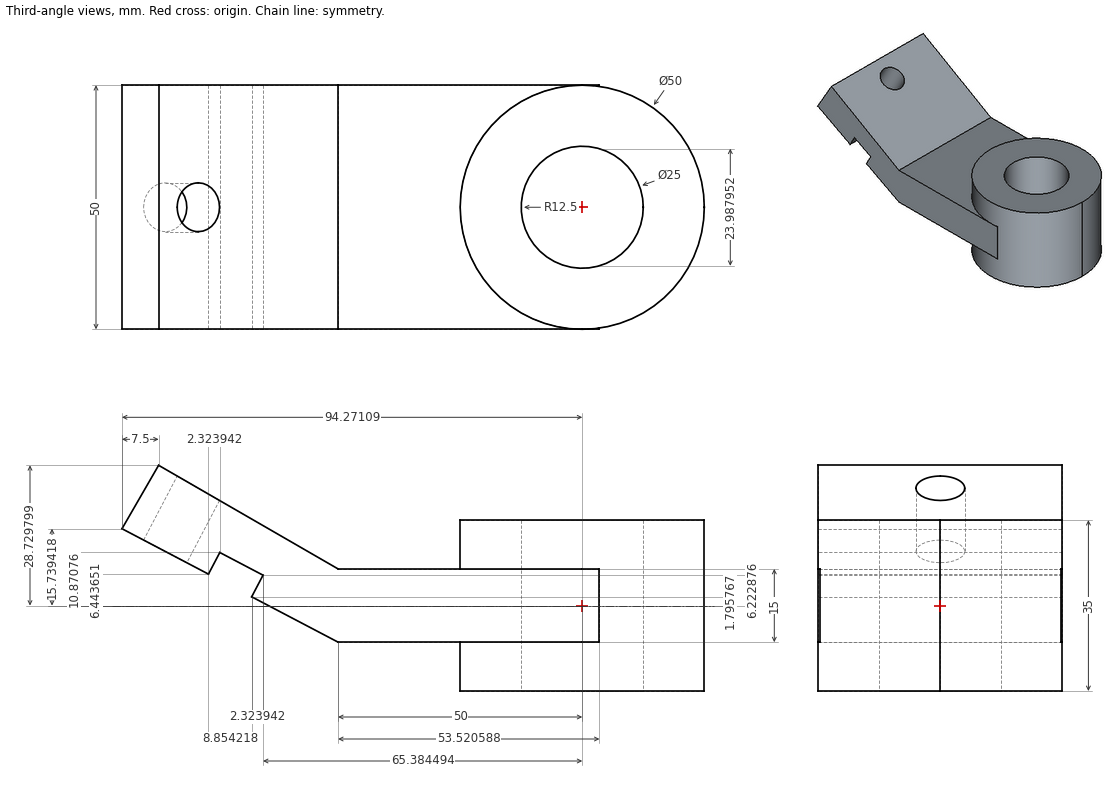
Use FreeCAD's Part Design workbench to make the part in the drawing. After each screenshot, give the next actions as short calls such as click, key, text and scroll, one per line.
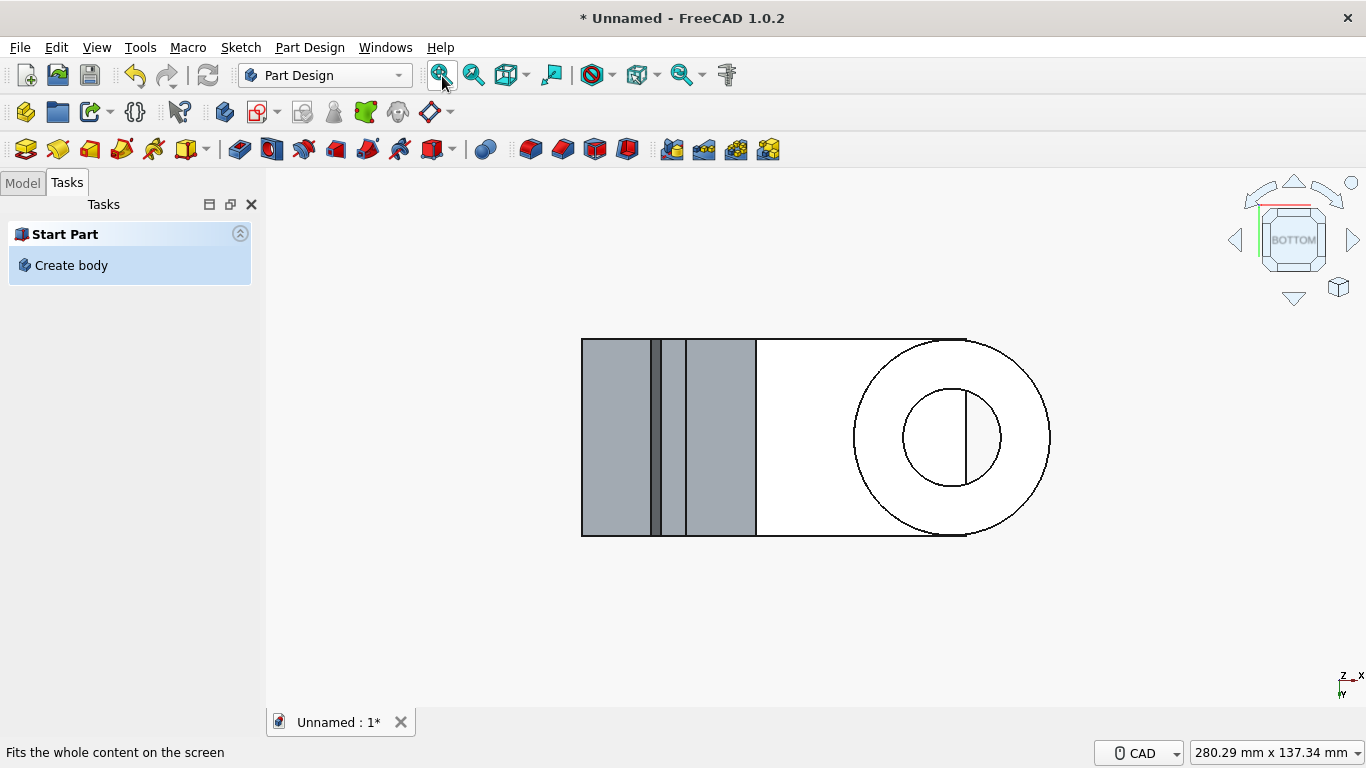
click(721, 493)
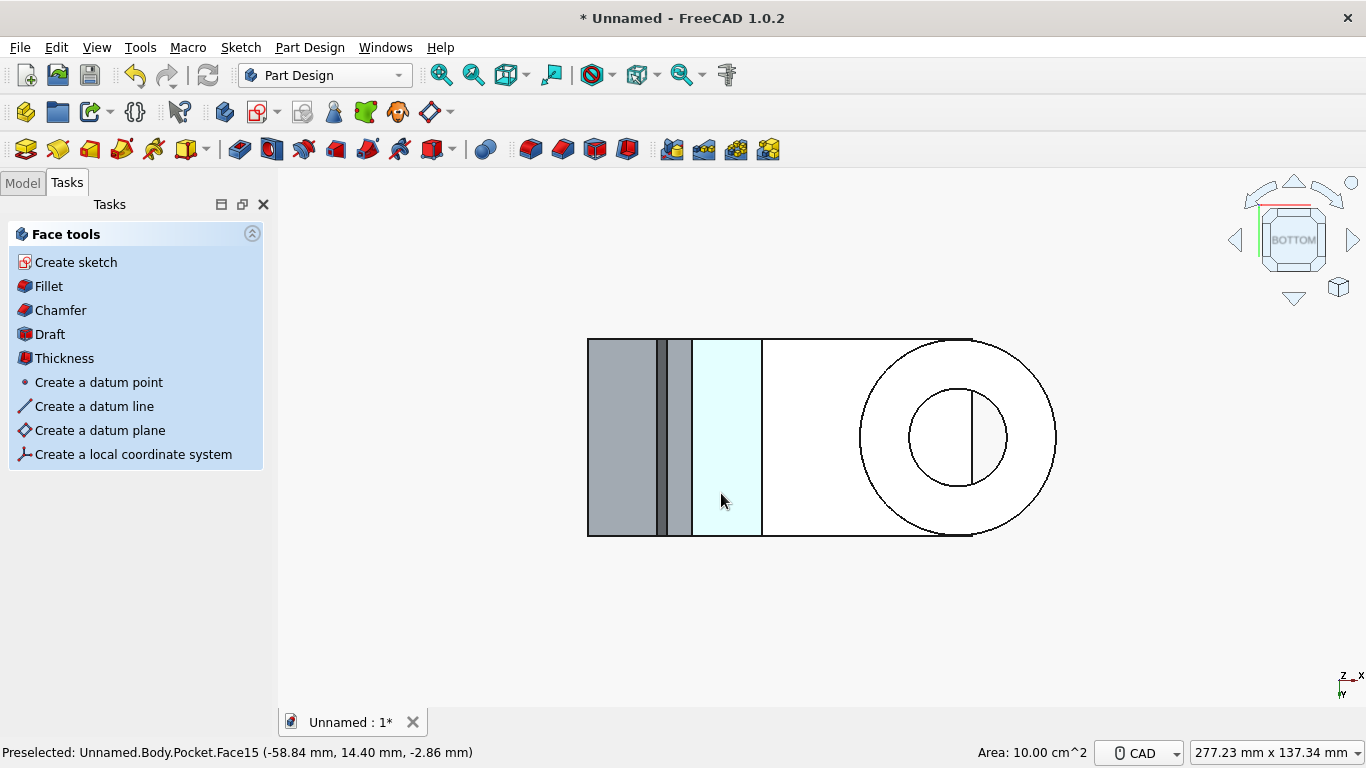
click(258, 112)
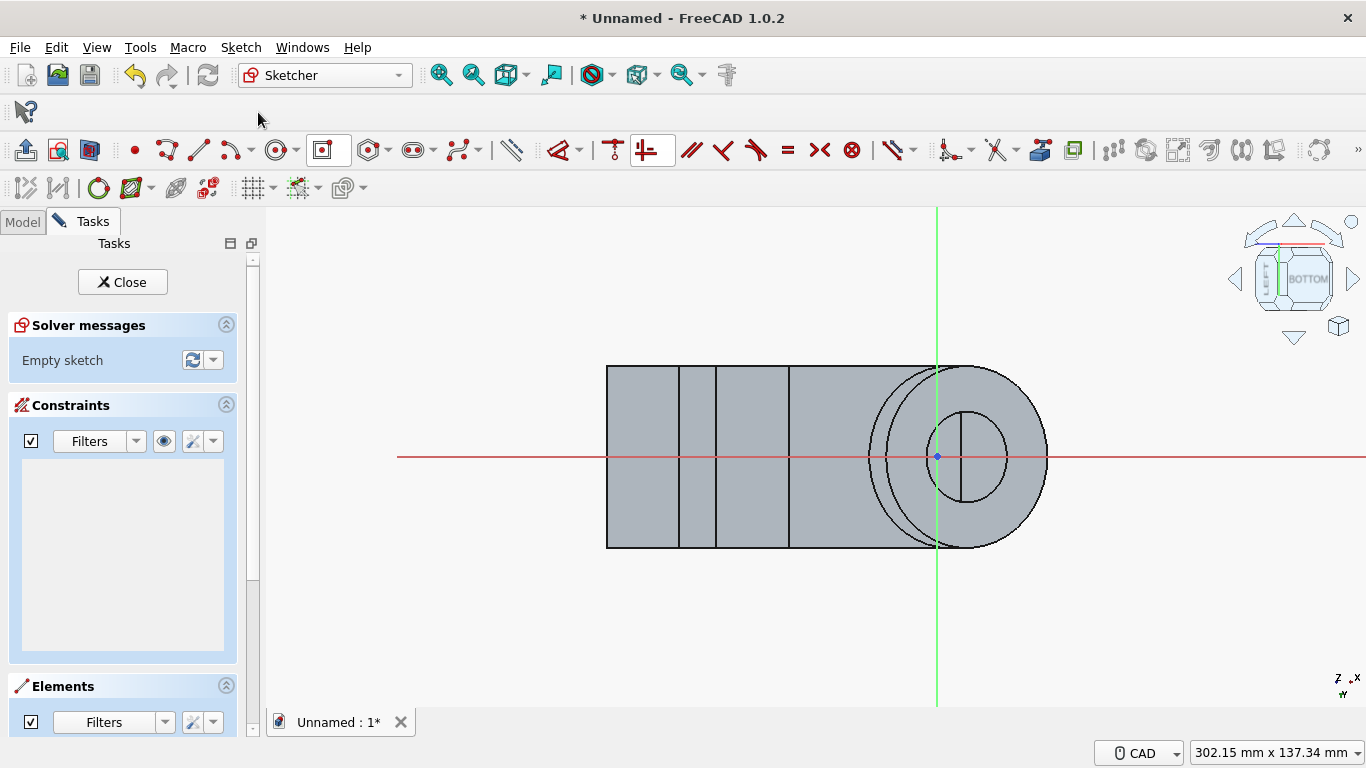
scroll(630, 457, up, 11)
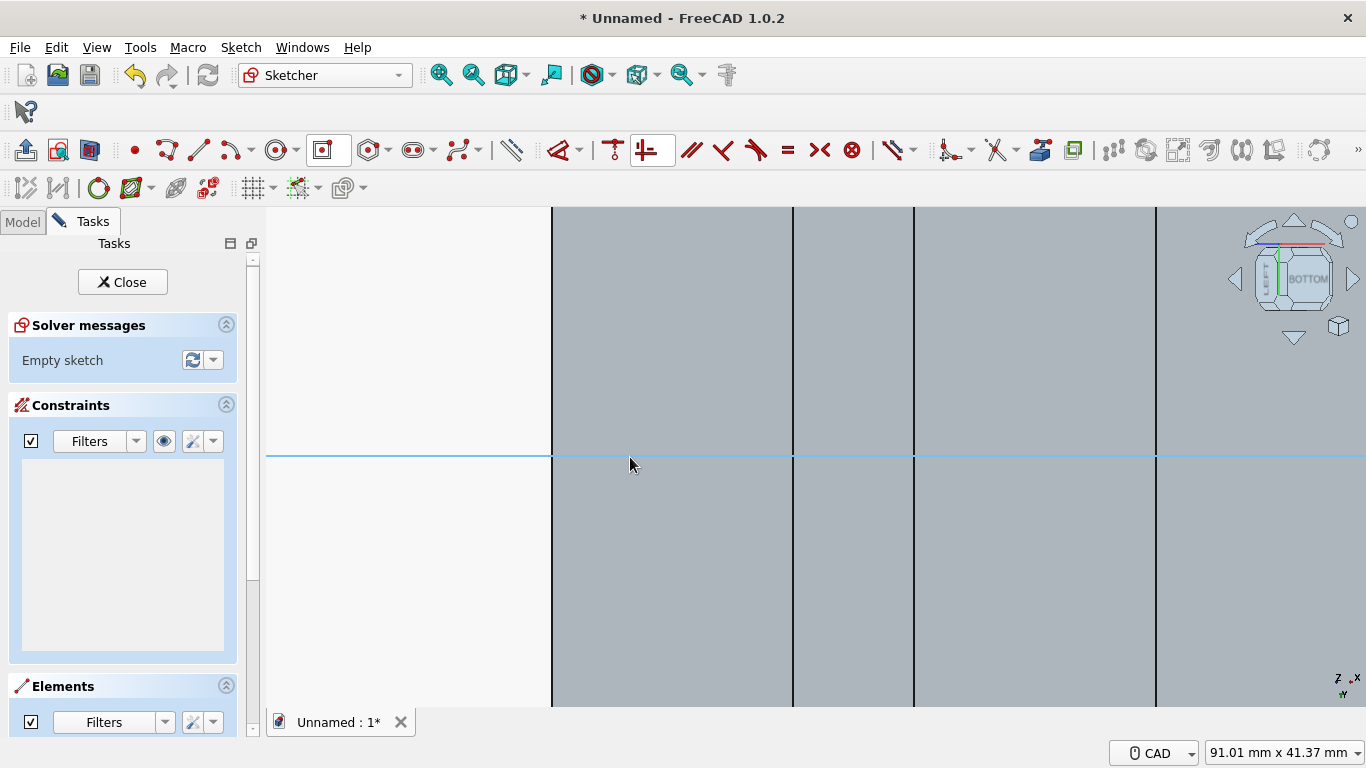
click(276, 150)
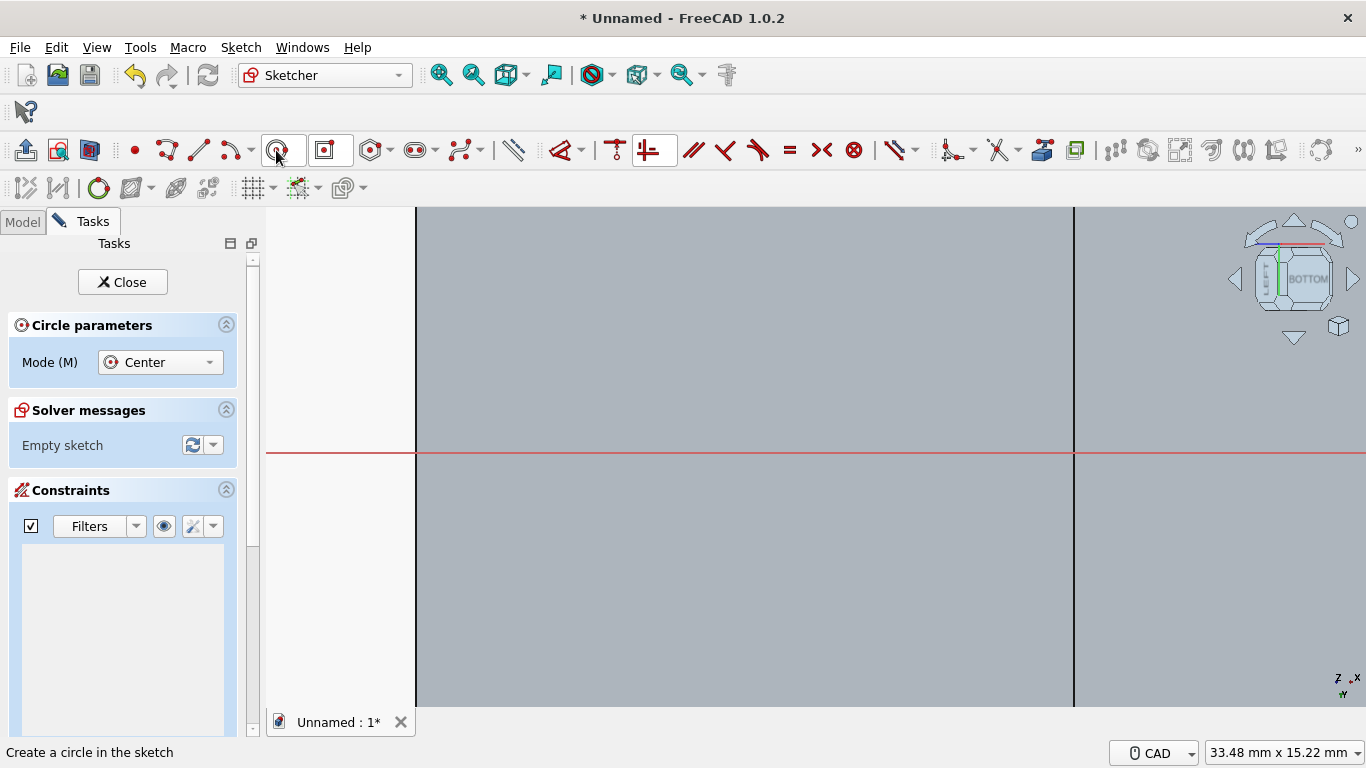
click(745, 453)
click(861, 337)
key(Escape)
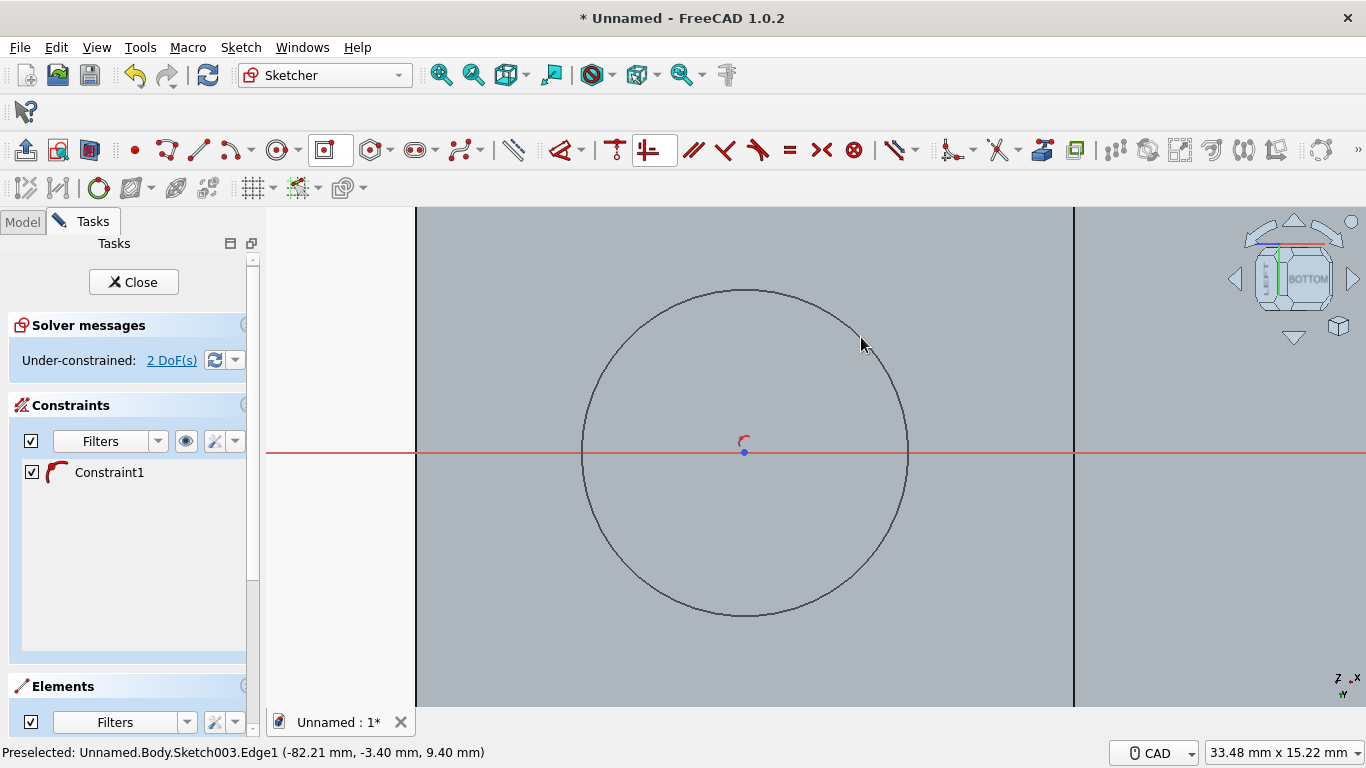
click(560, 150)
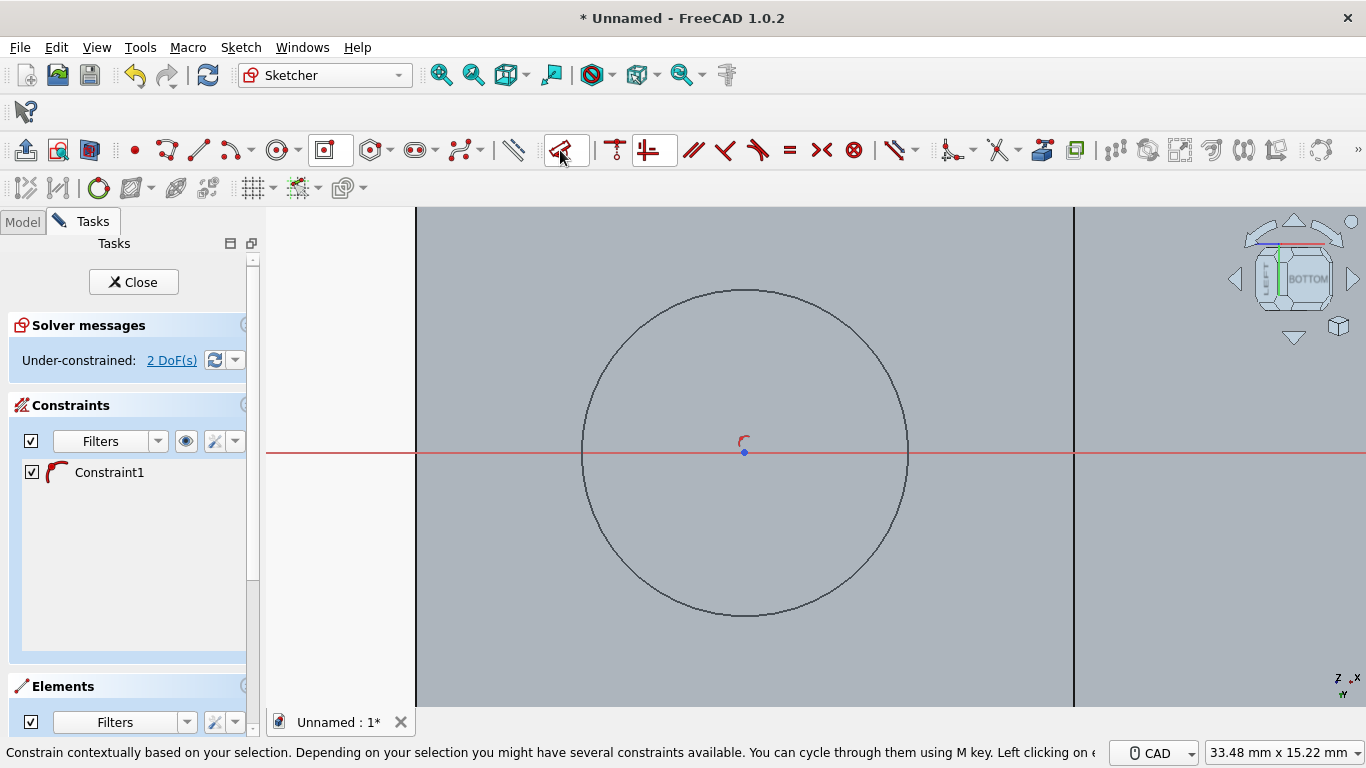
click(860, 337)
click(883, 314)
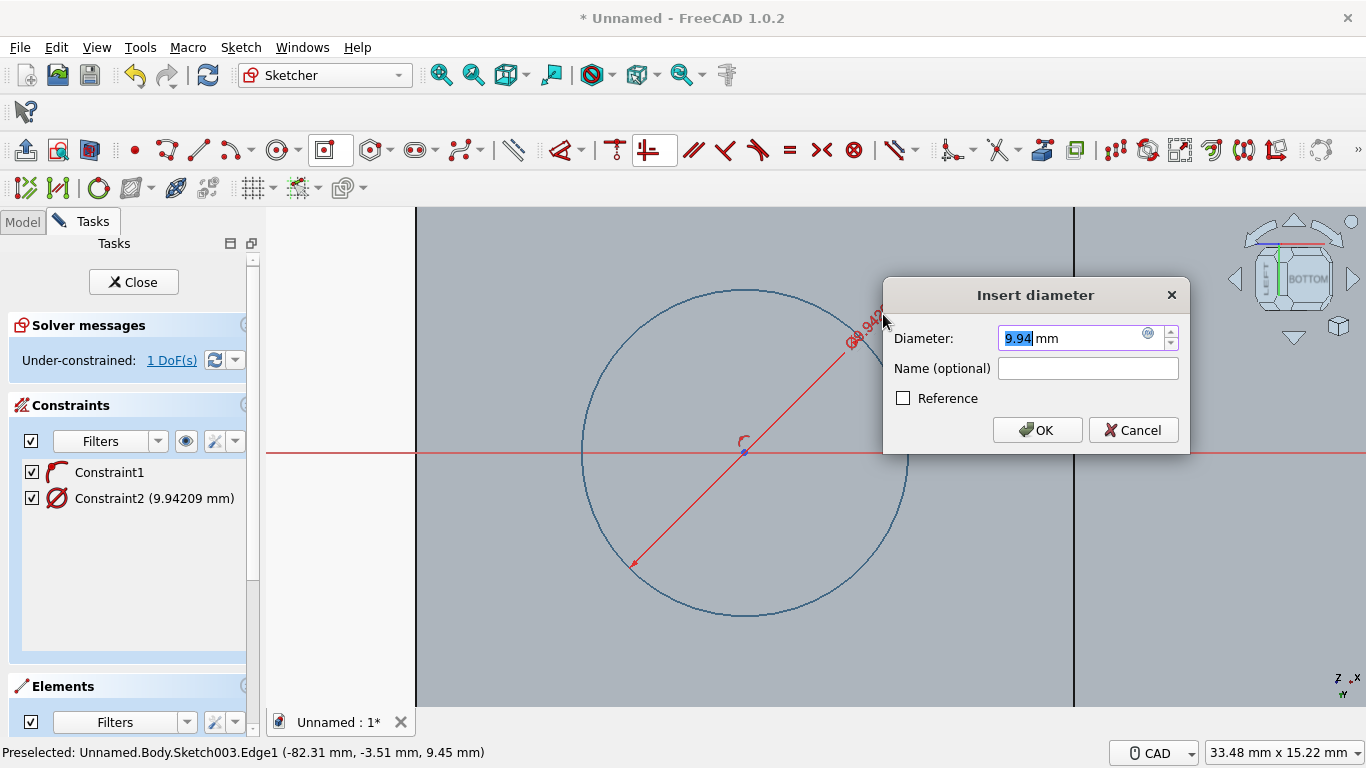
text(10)
key(Return)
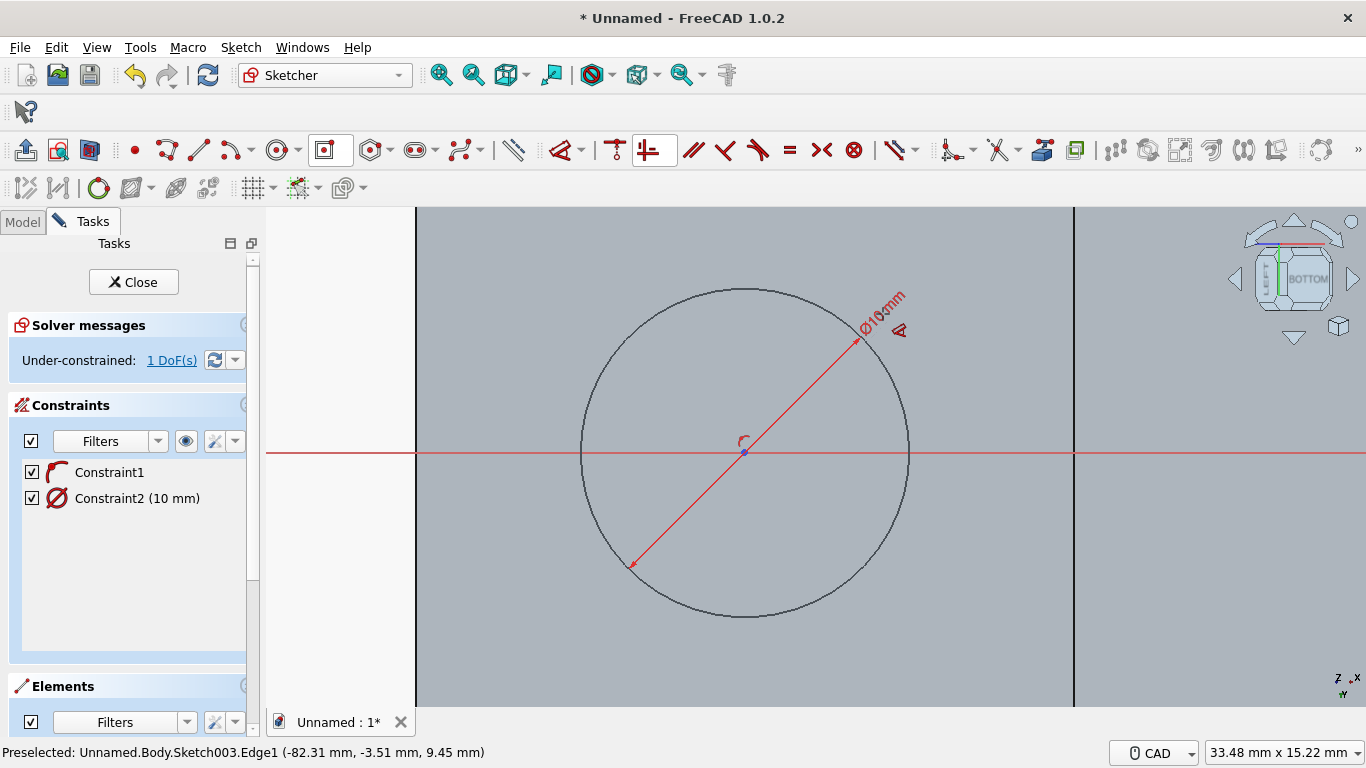
click(745, 453)
click(973, 487)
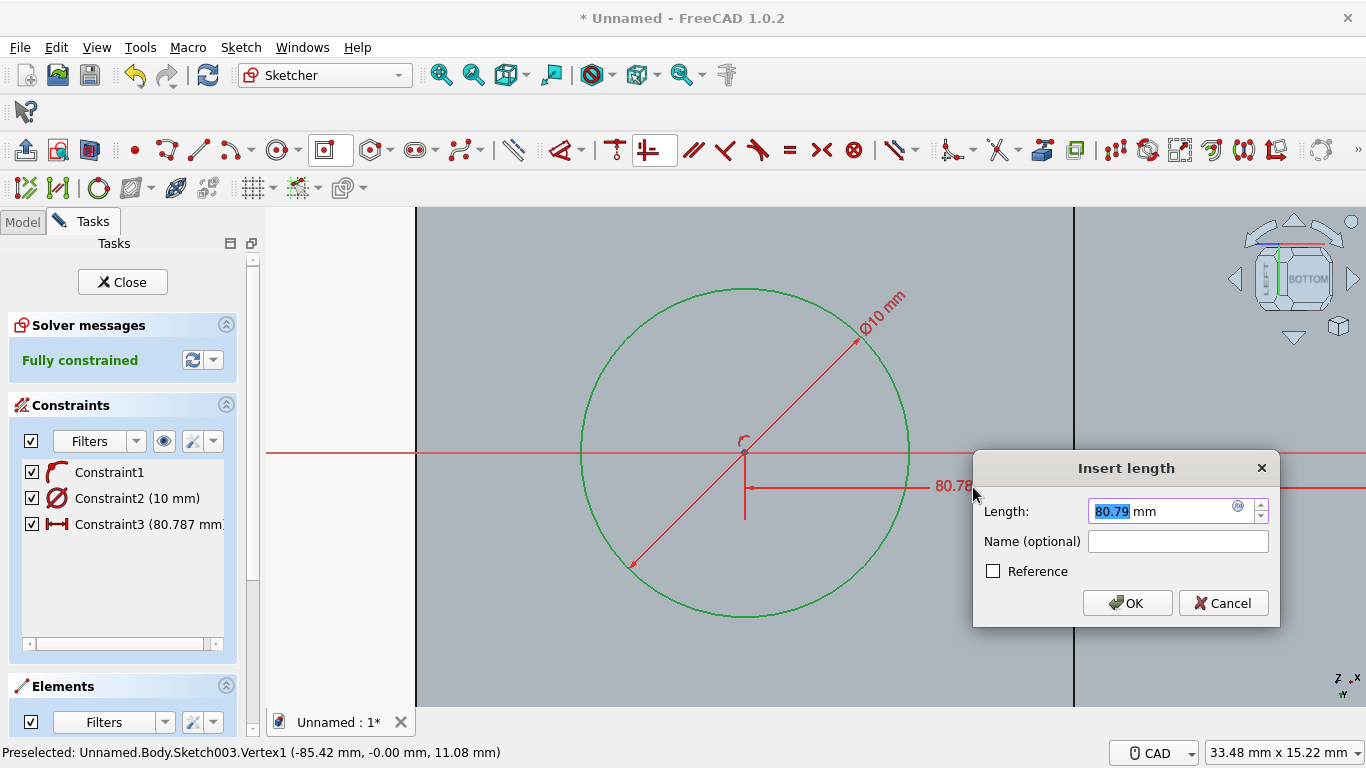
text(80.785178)
key(Return)
key(Escape)